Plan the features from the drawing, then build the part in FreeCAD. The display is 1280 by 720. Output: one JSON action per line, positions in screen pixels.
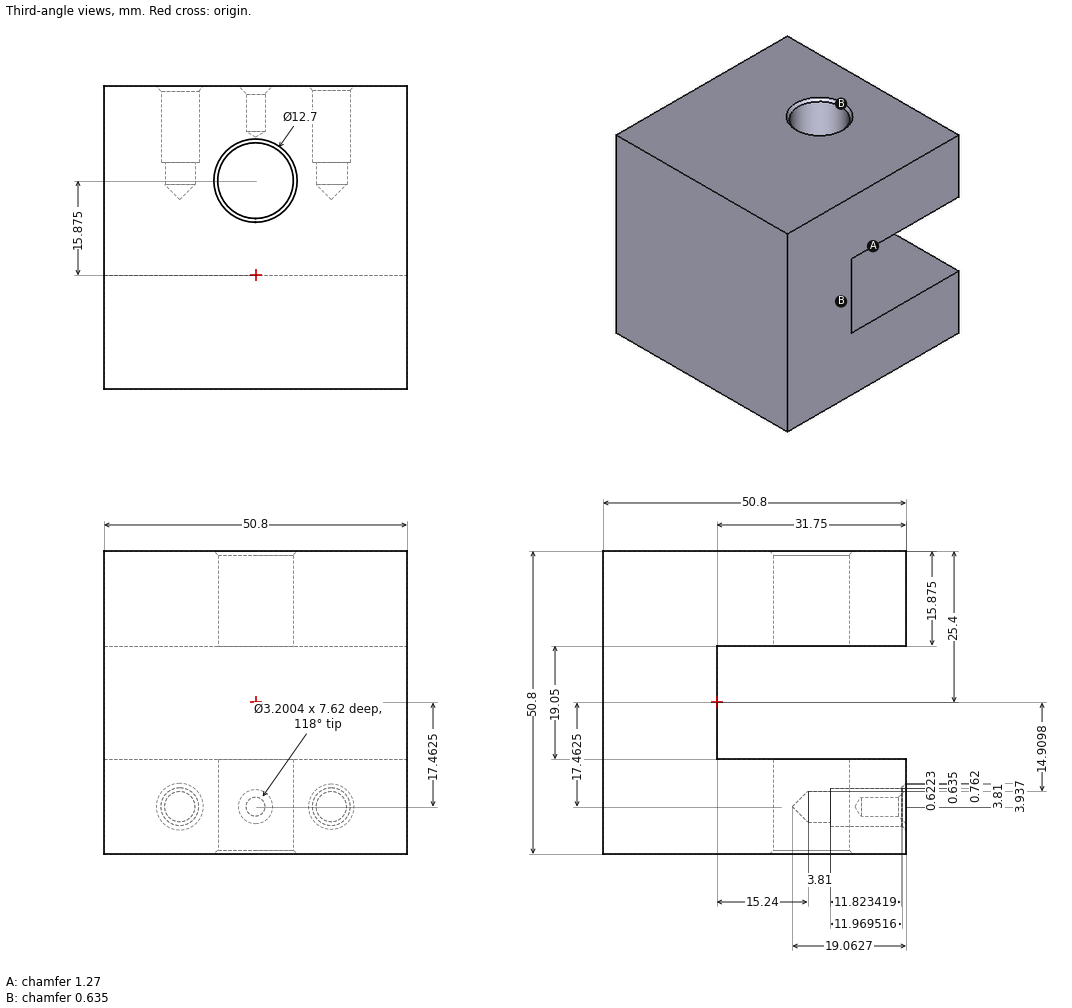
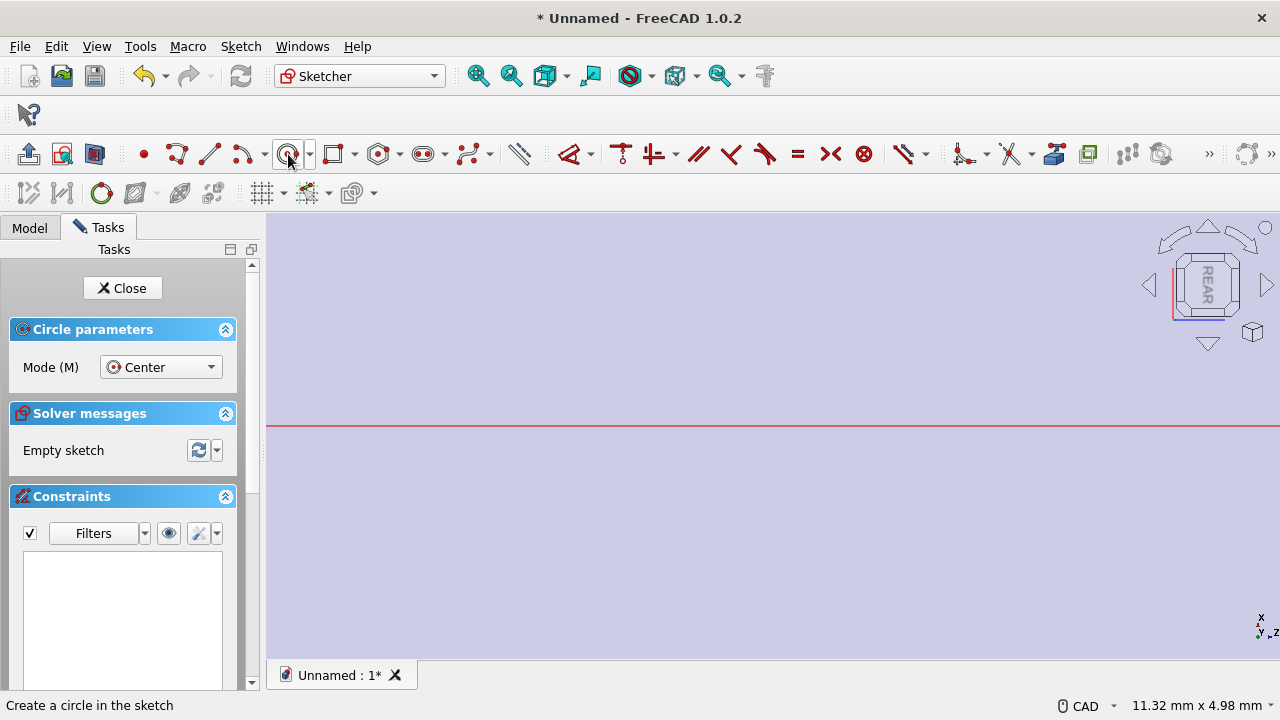
{"action": "left_click", "coordinate": [689, 426]}
{"action": "left_click", "coordinate": [791, 325]}
{"action": "key", "text": "Escape"}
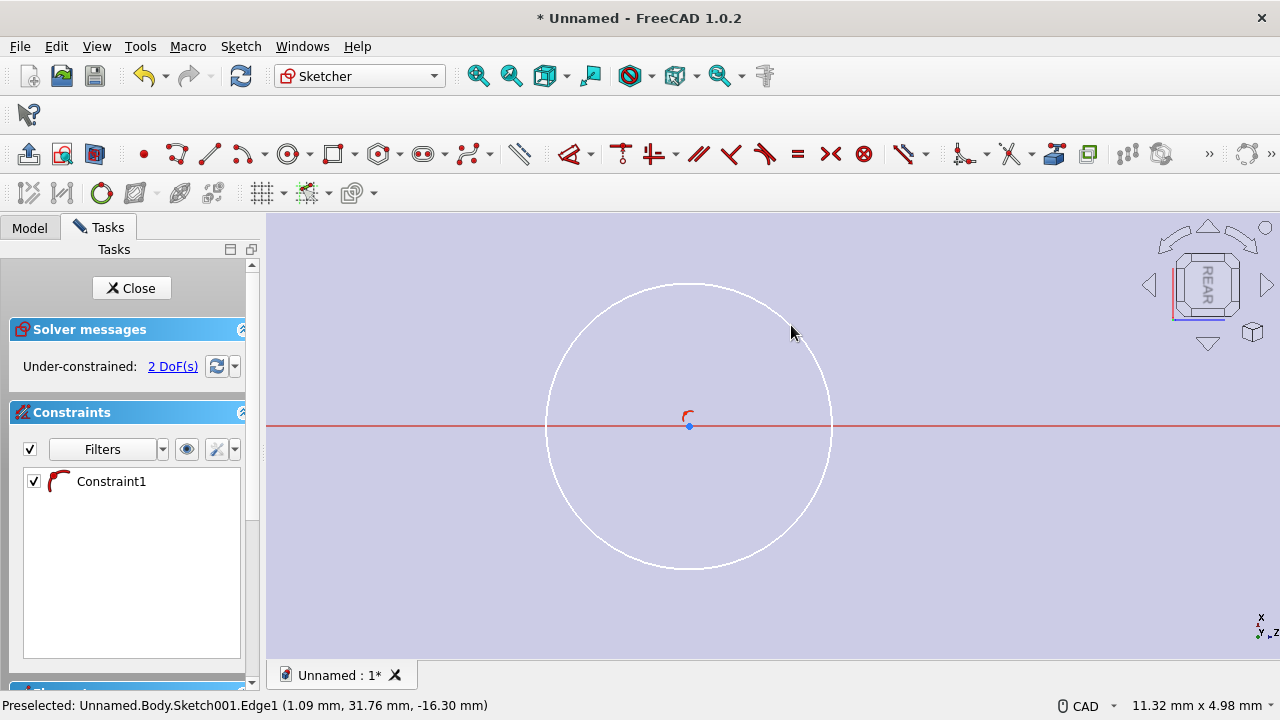
{"action": "left_click", "coordinate": [568, 154]}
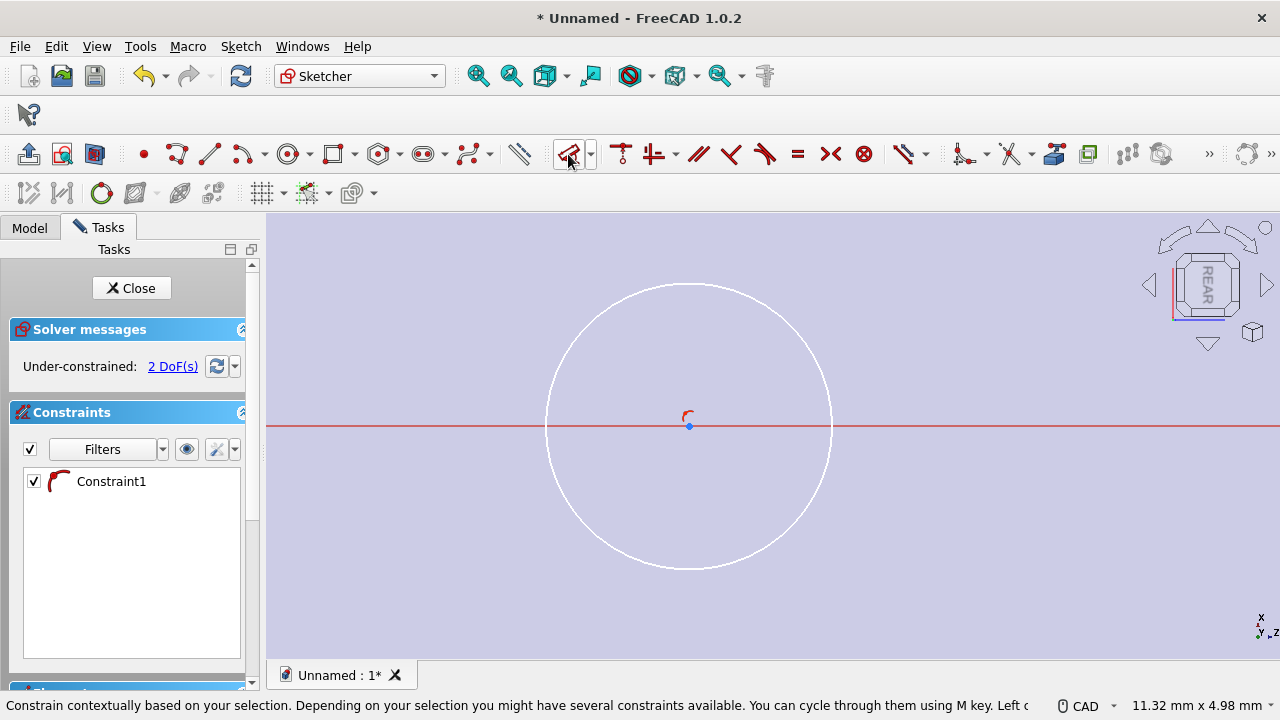
{"action": "left_click", "coordinate": [790, 325]}
{"action": "left_click", "coordinate": [813, 302]}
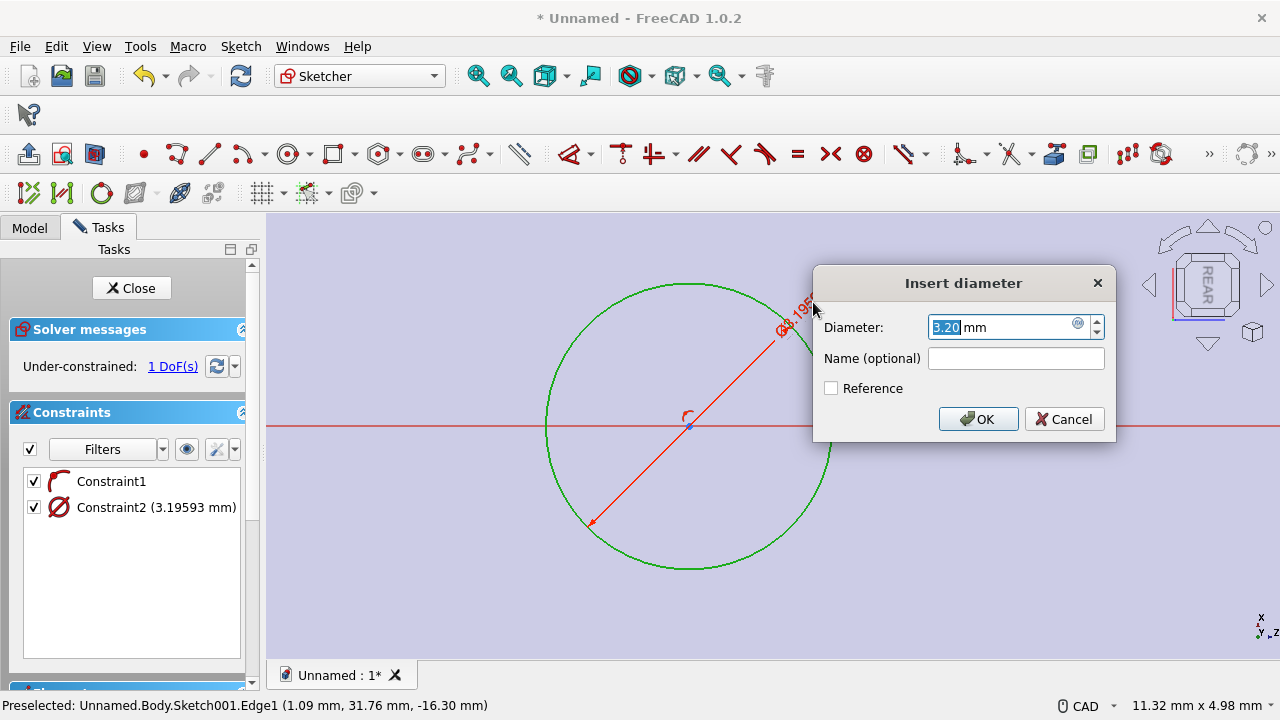
{"action": "type", "text": "3.2004"}
{"action": "key", "text": "Return"}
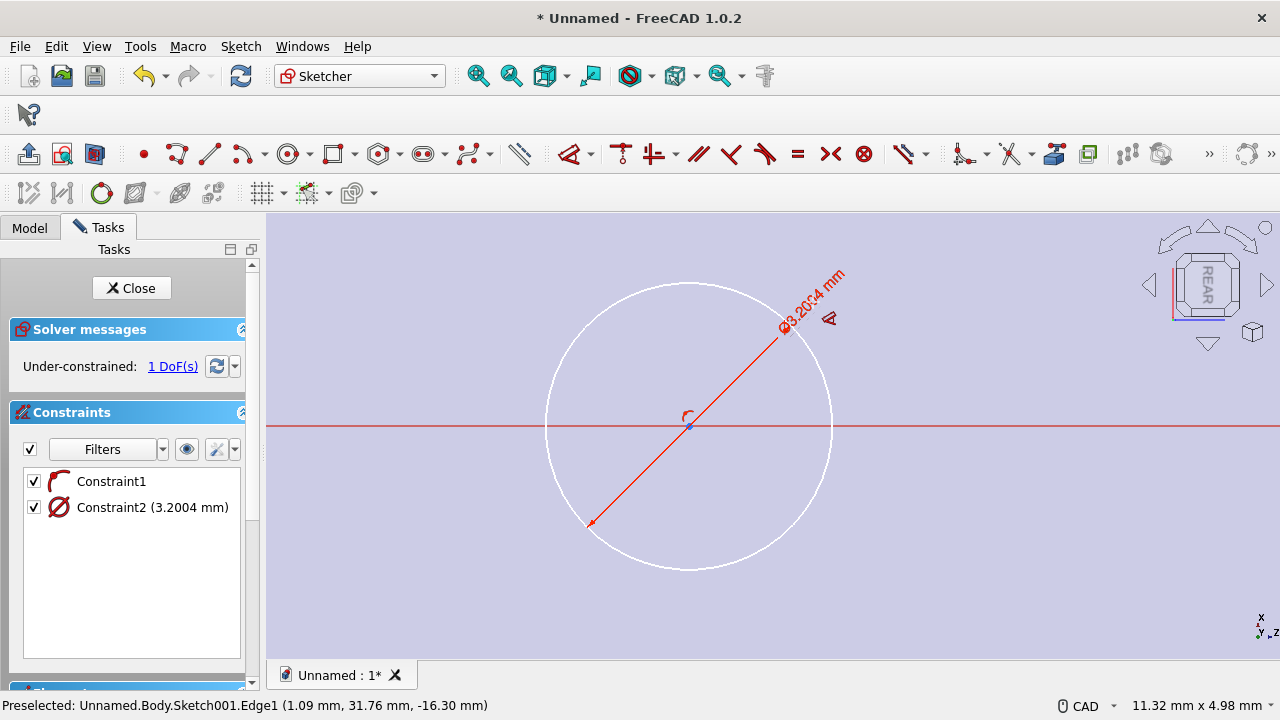
{"action": "left_click", "coordinate": [689, 426]}
{"action": "left_click", "coordinate": [902, 460]}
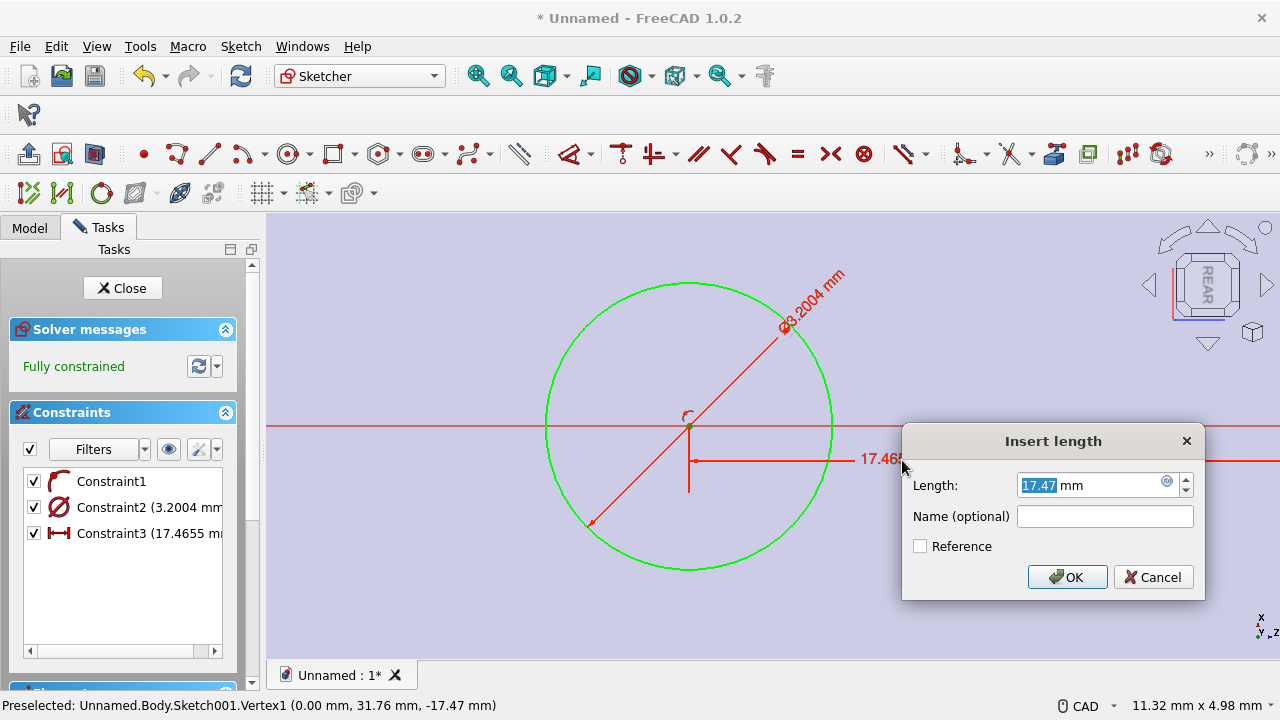
{"action": "type", "text": "17.4625"}
{"action": "key", "text": "Return"}
{"action": "key", "text": "Escape"}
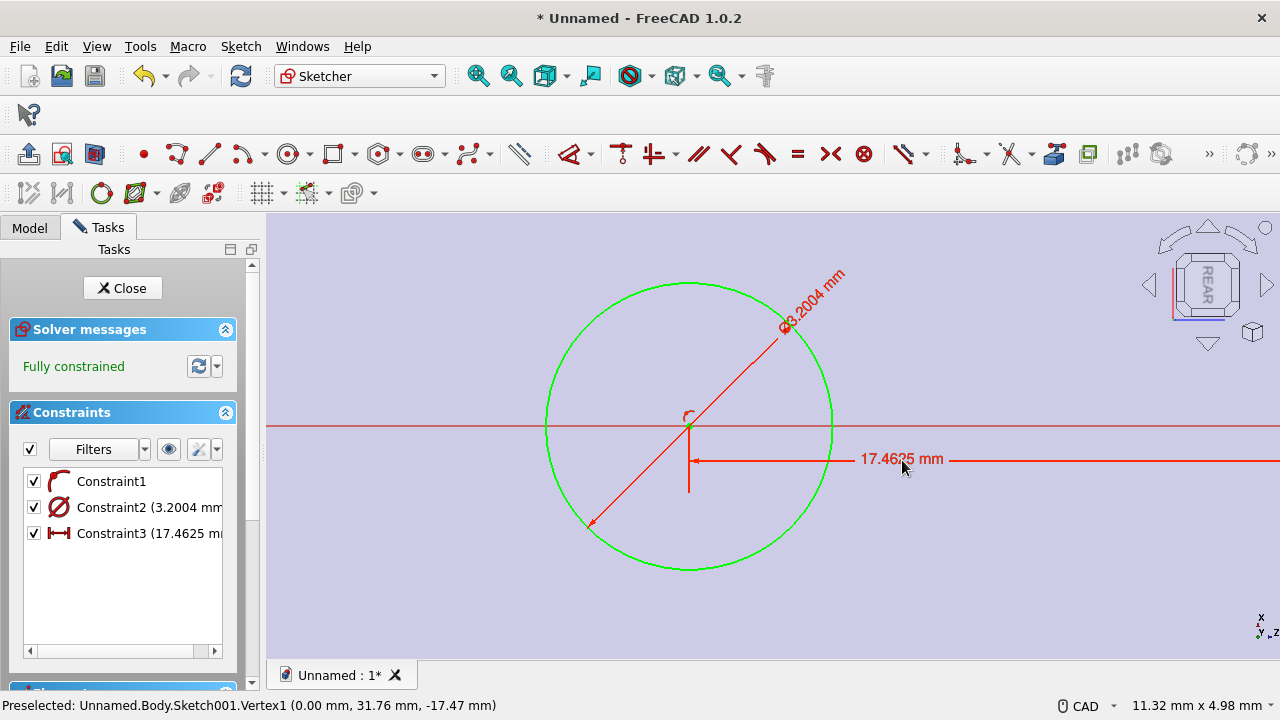
{"action": "left_click", "coordinate": [123, 288]}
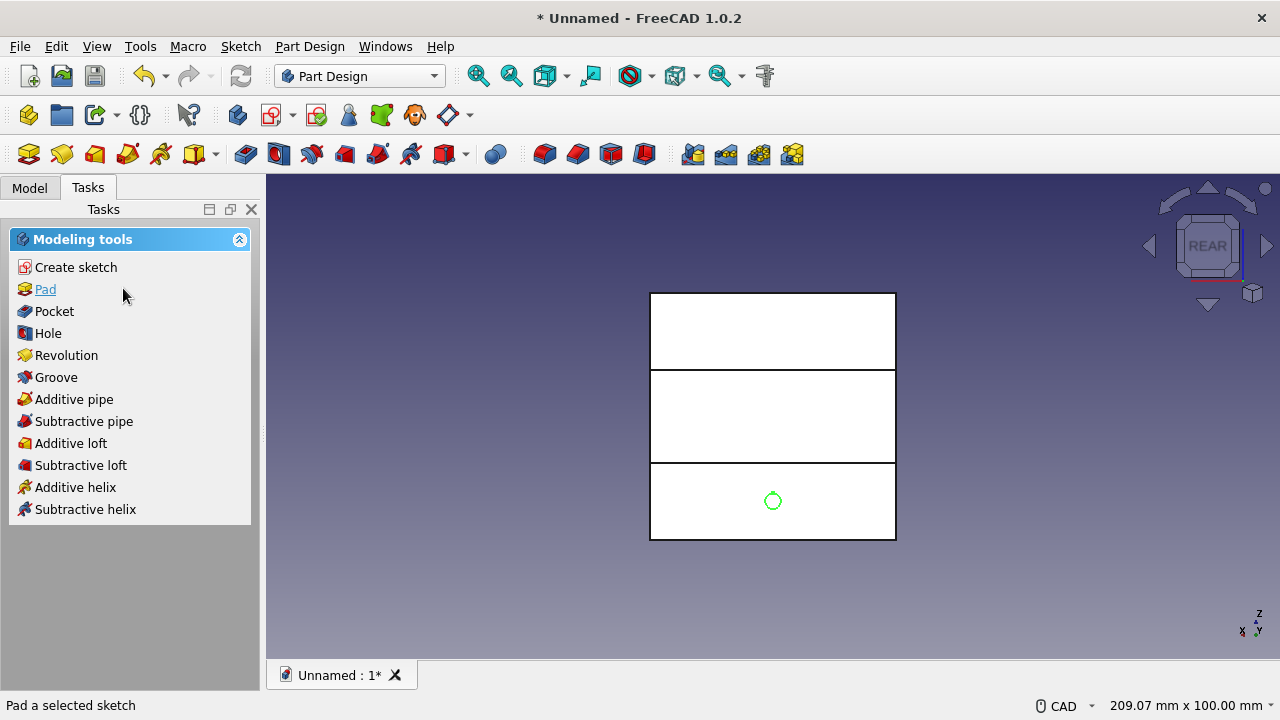
{"action": "left_click", "coordinate": [279, 154]}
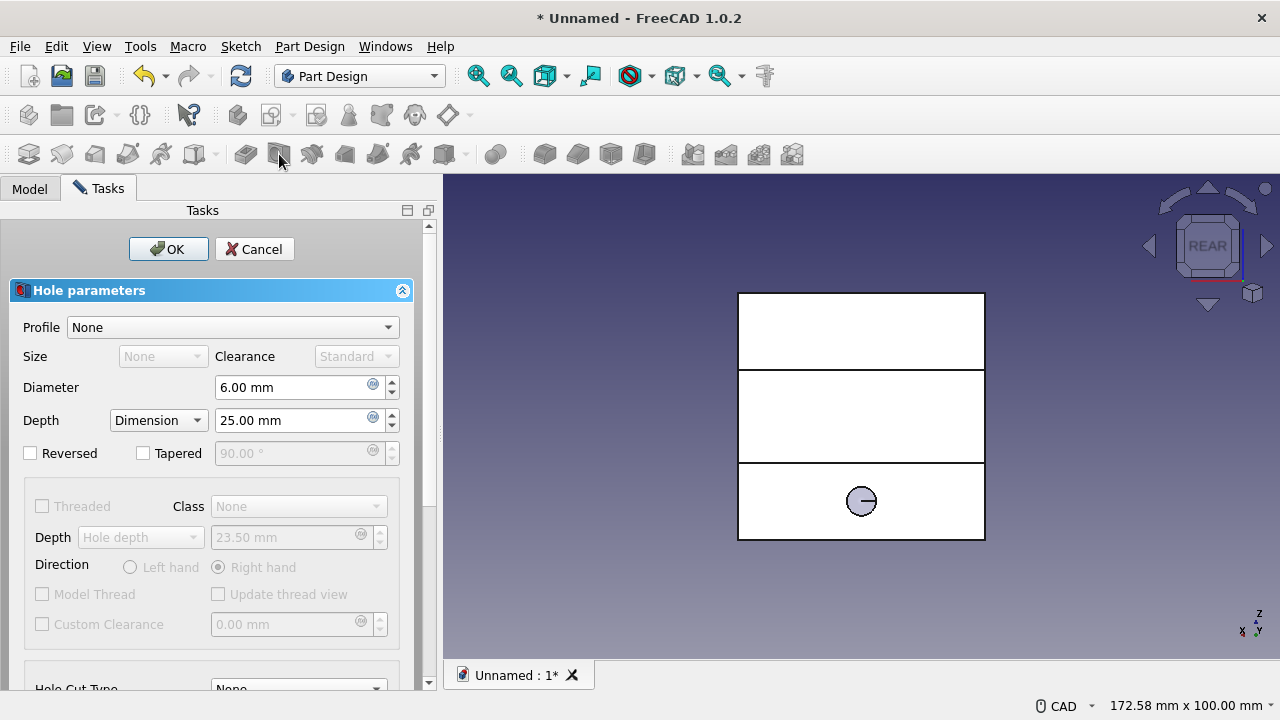
{"action": "triple_click", "coordinate": [300, 388]}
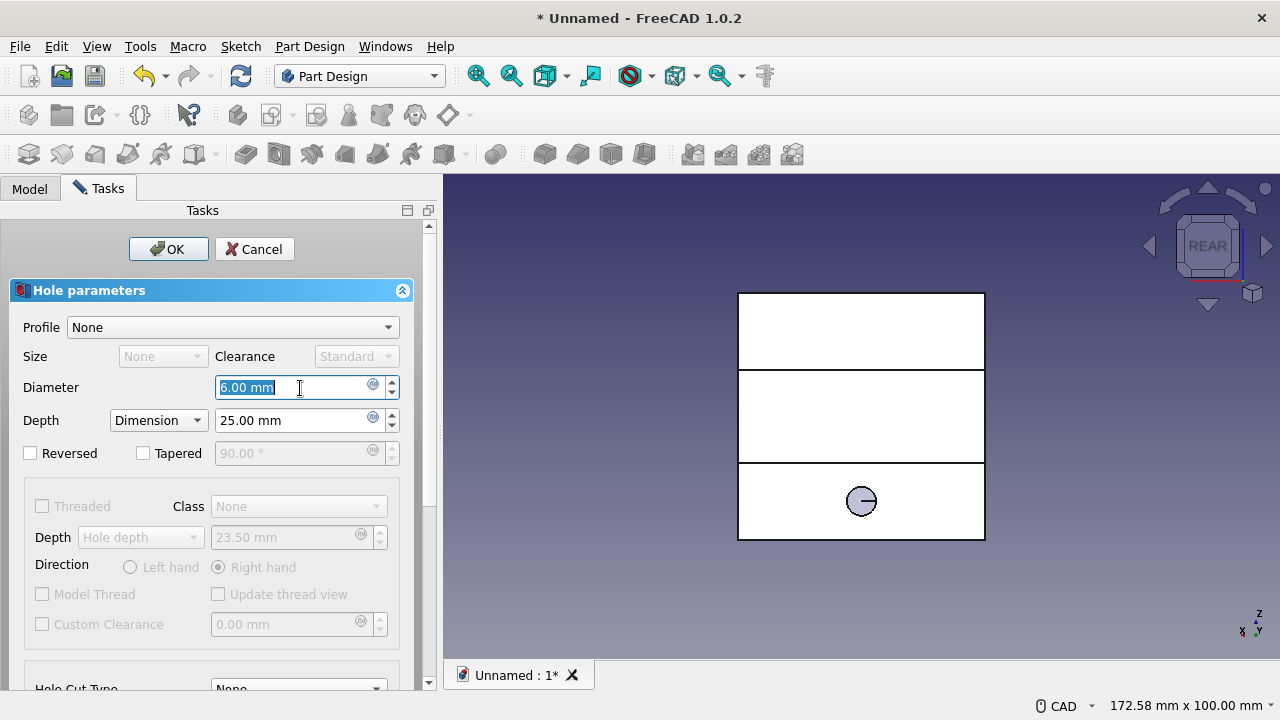
{"action": "type", "text": "3.2004"}
{"action": "key", "text": "Tab"}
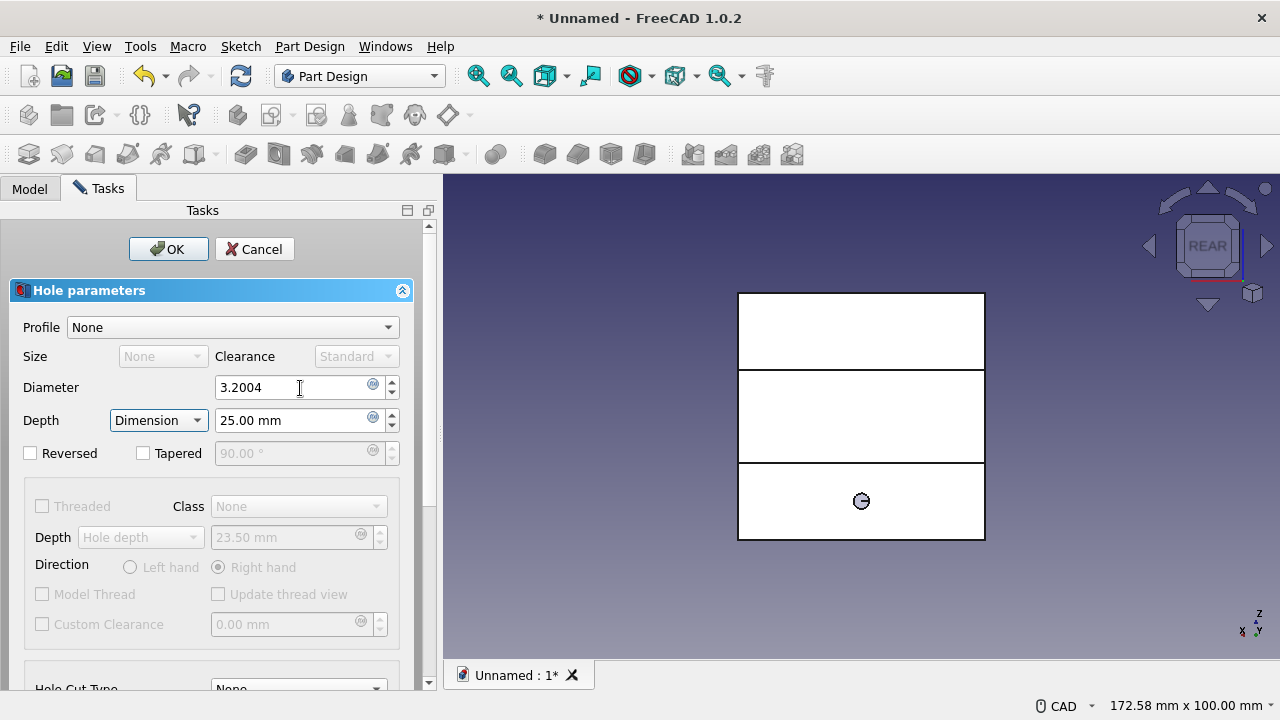
{"action": "triple_click", "coordinate": [300, 420]}